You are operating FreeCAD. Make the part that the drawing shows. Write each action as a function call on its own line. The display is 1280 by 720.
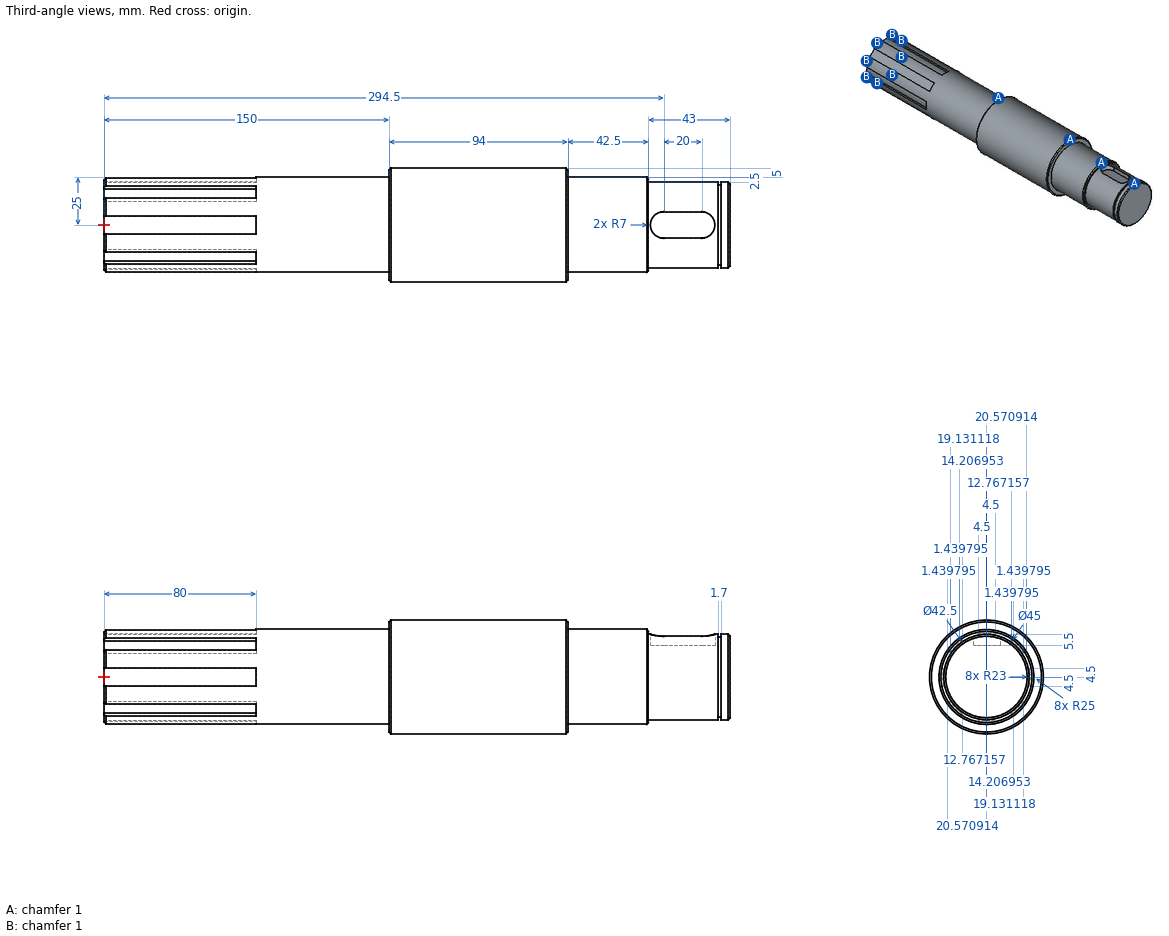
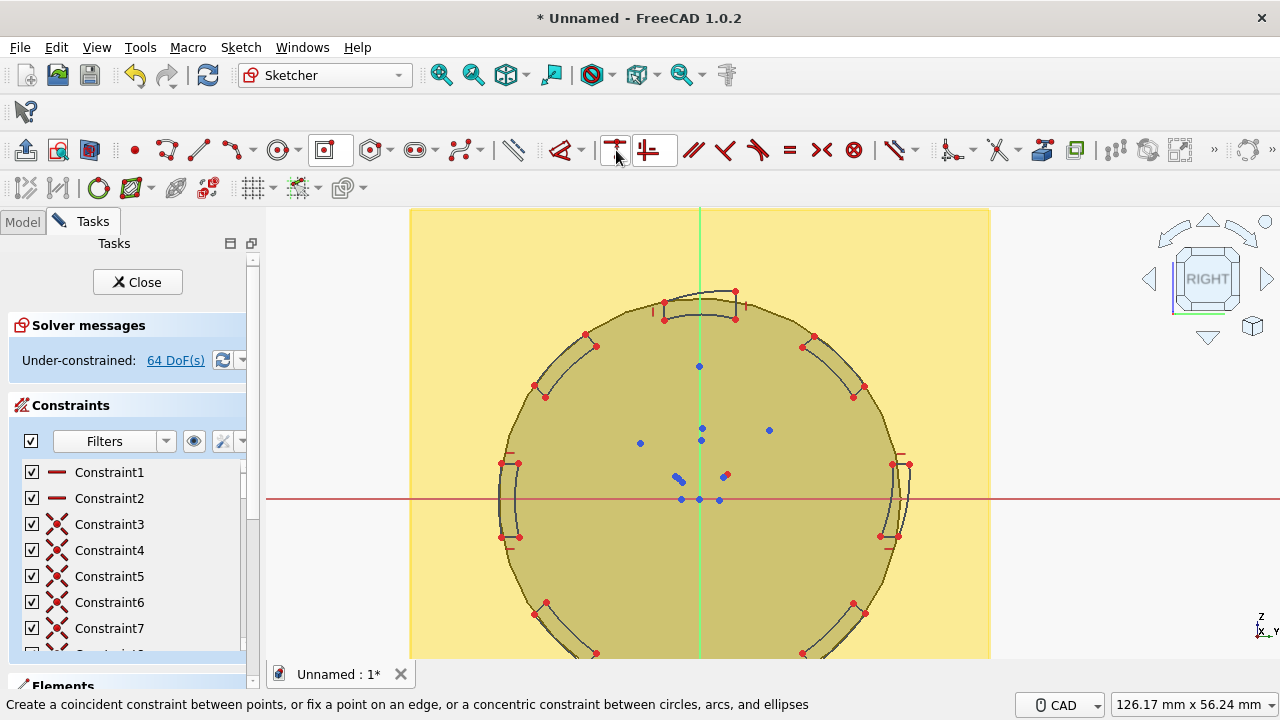
click(888, 516)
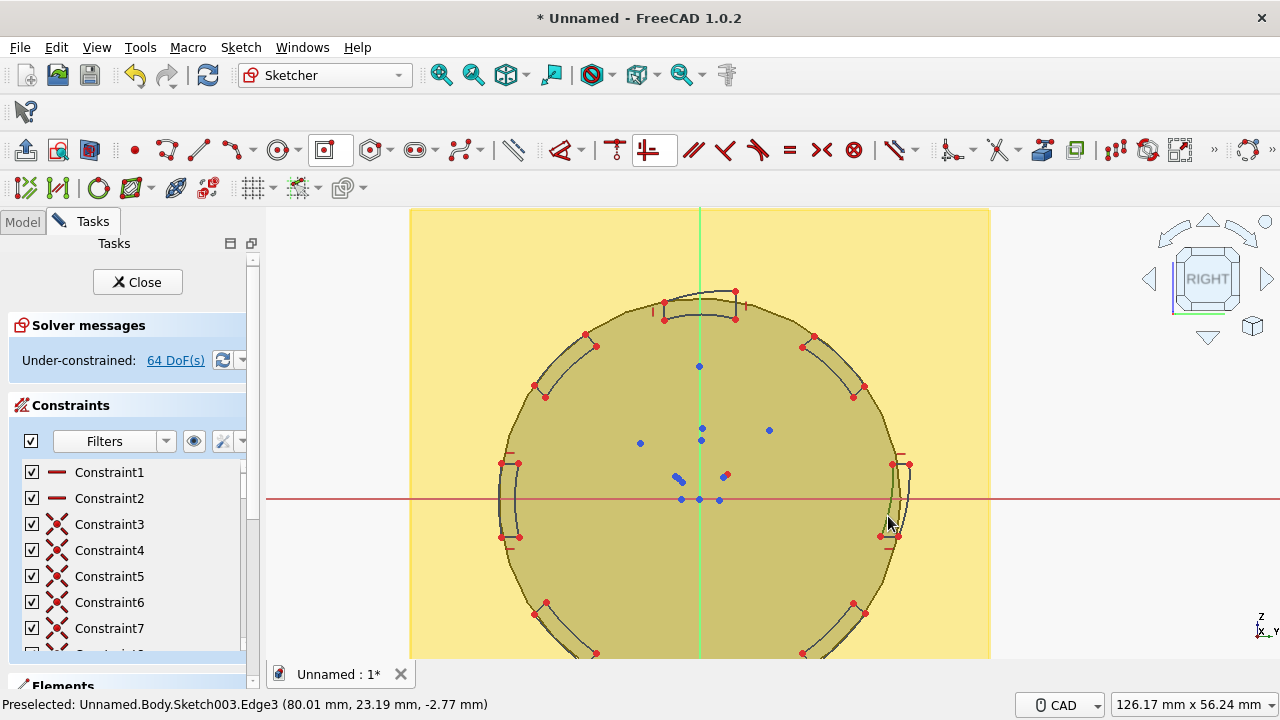
click(714, 315)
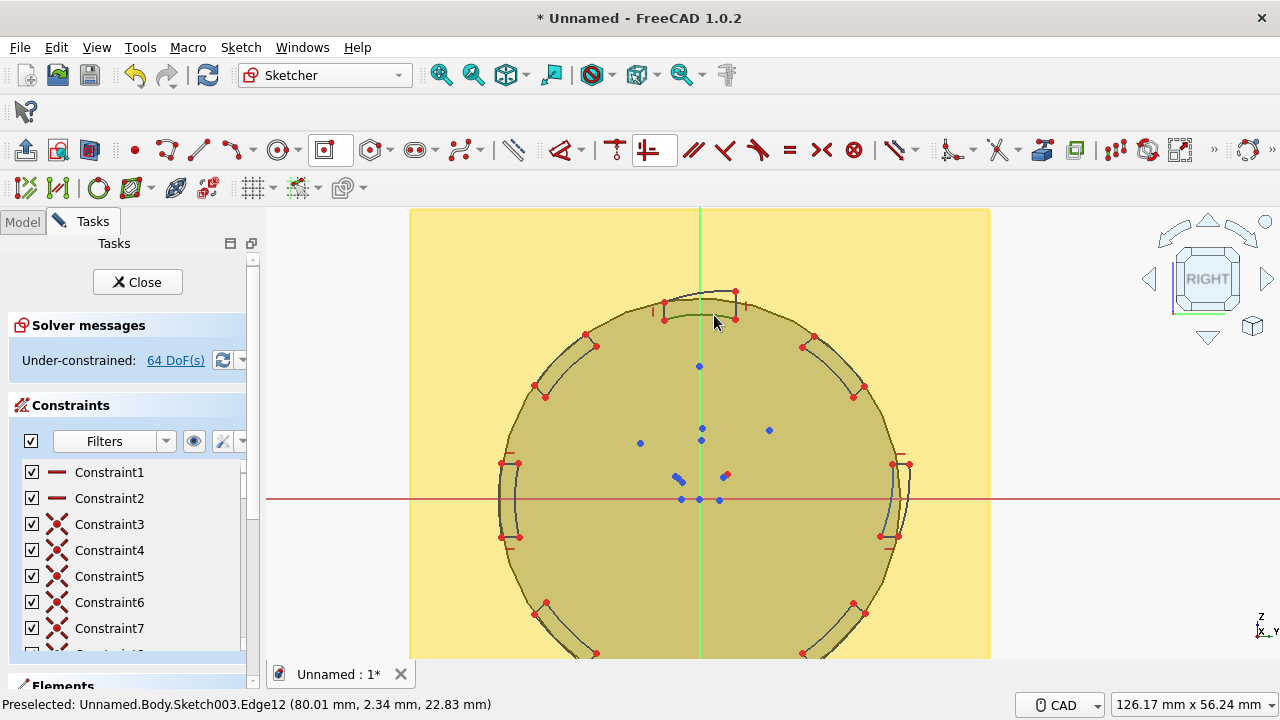
click(616, 150)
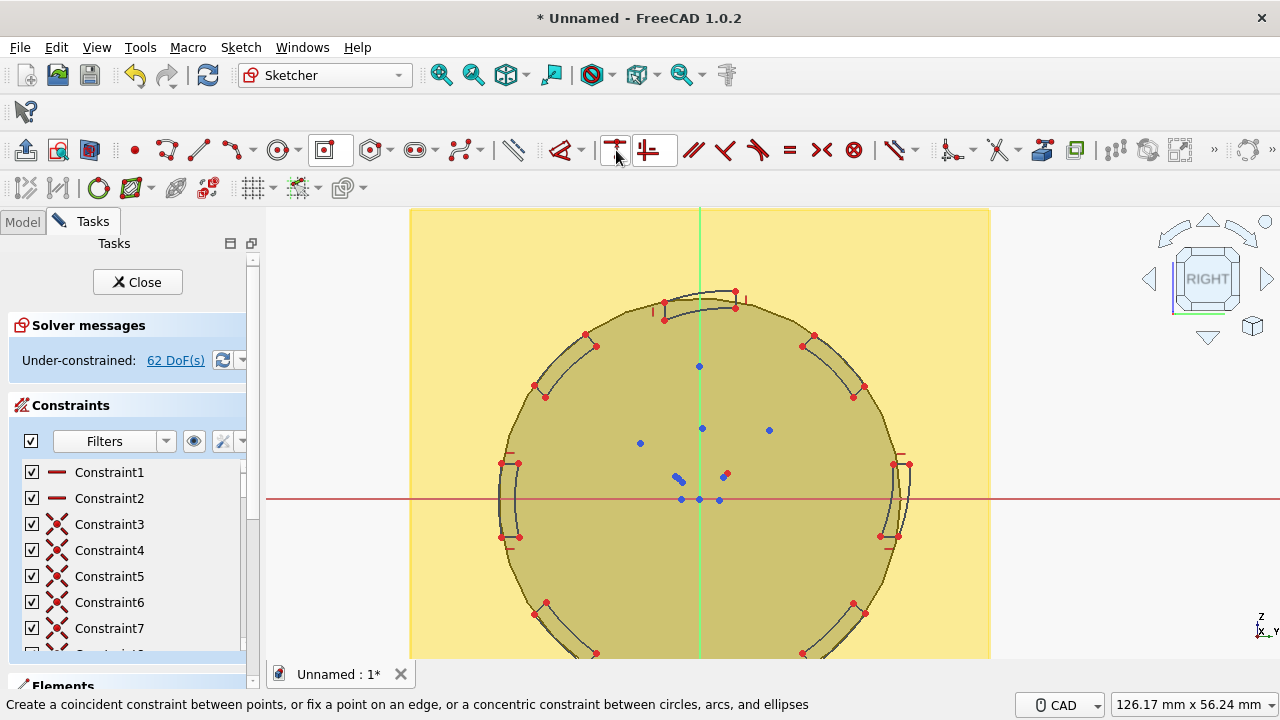
click(888, 516)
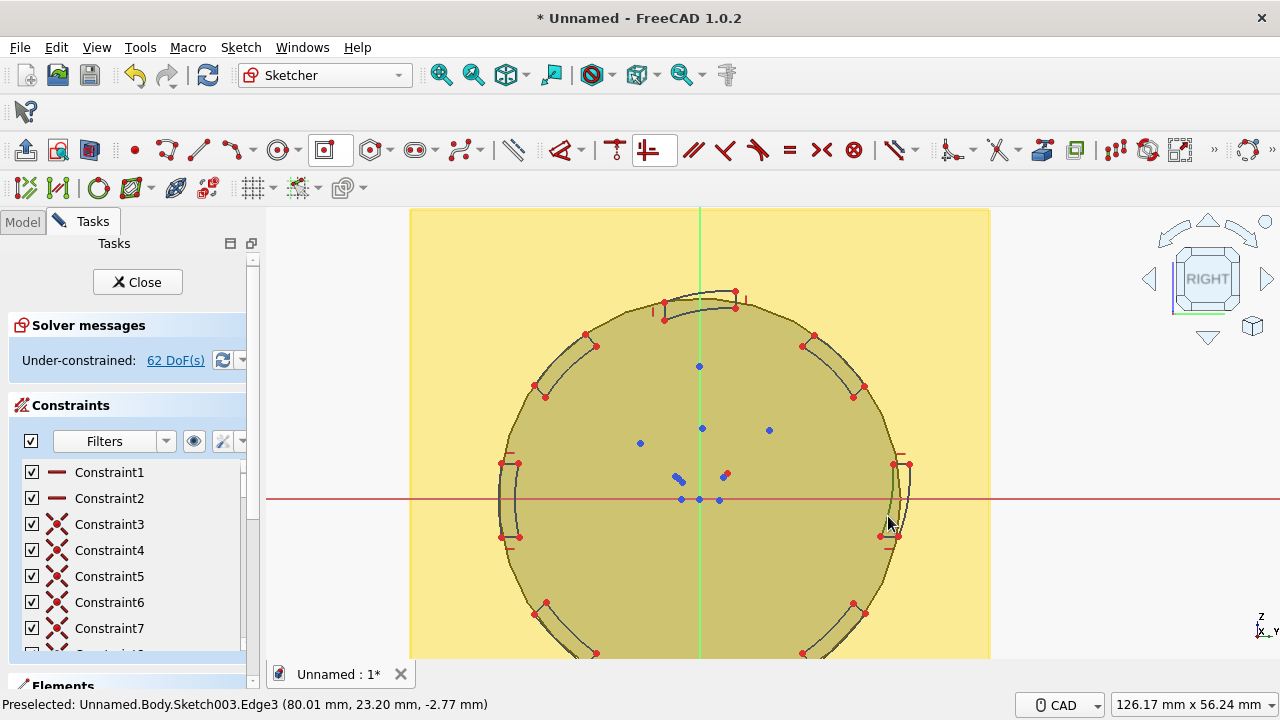
click(568, 347)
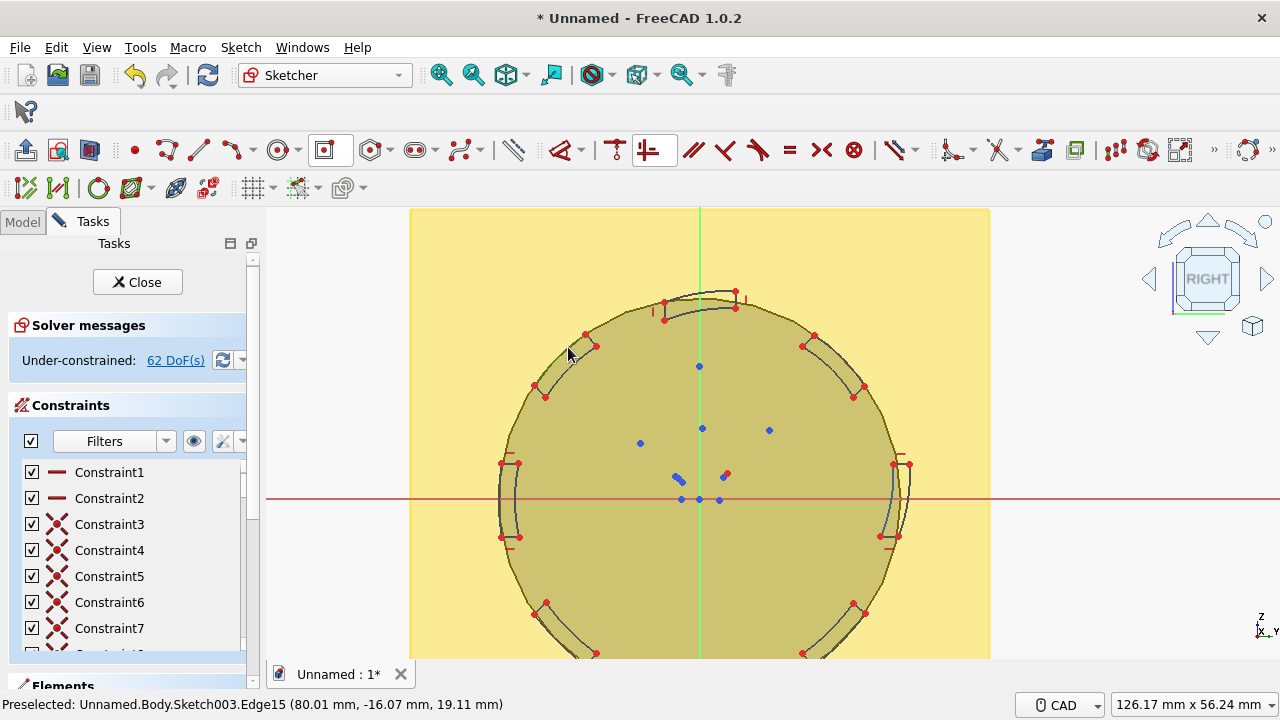
click(616, 150)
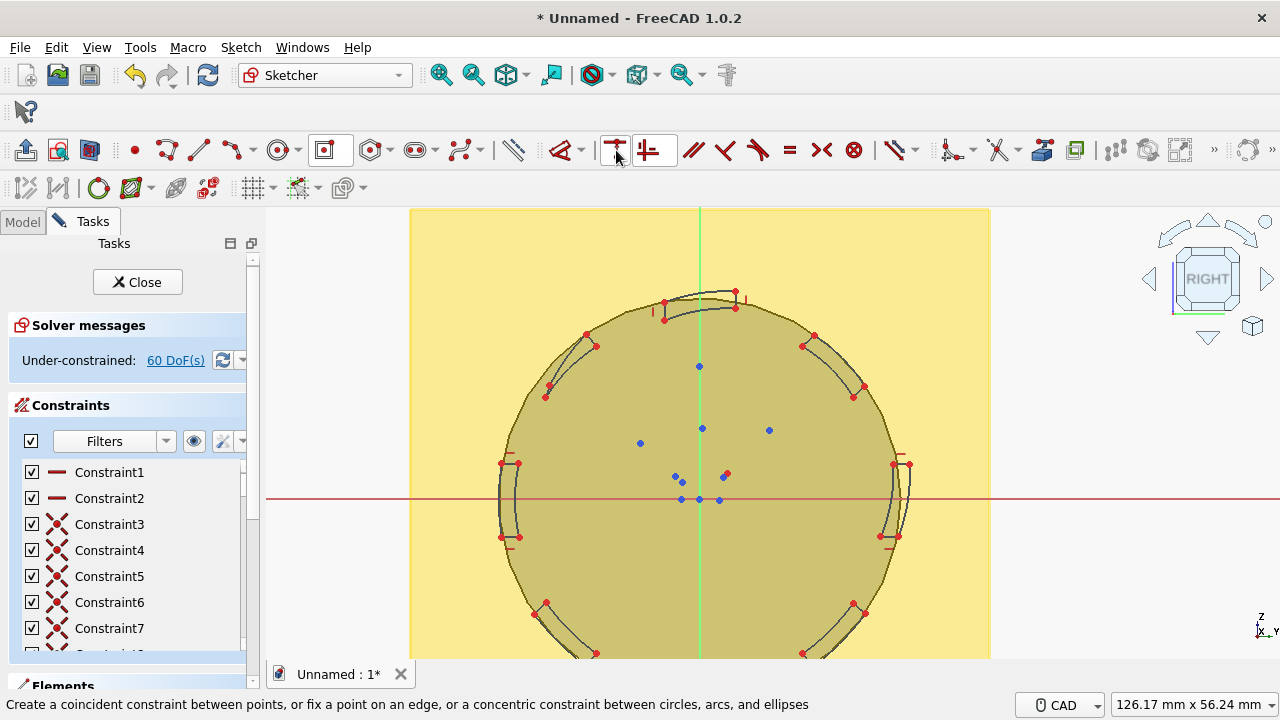
click(888, 516)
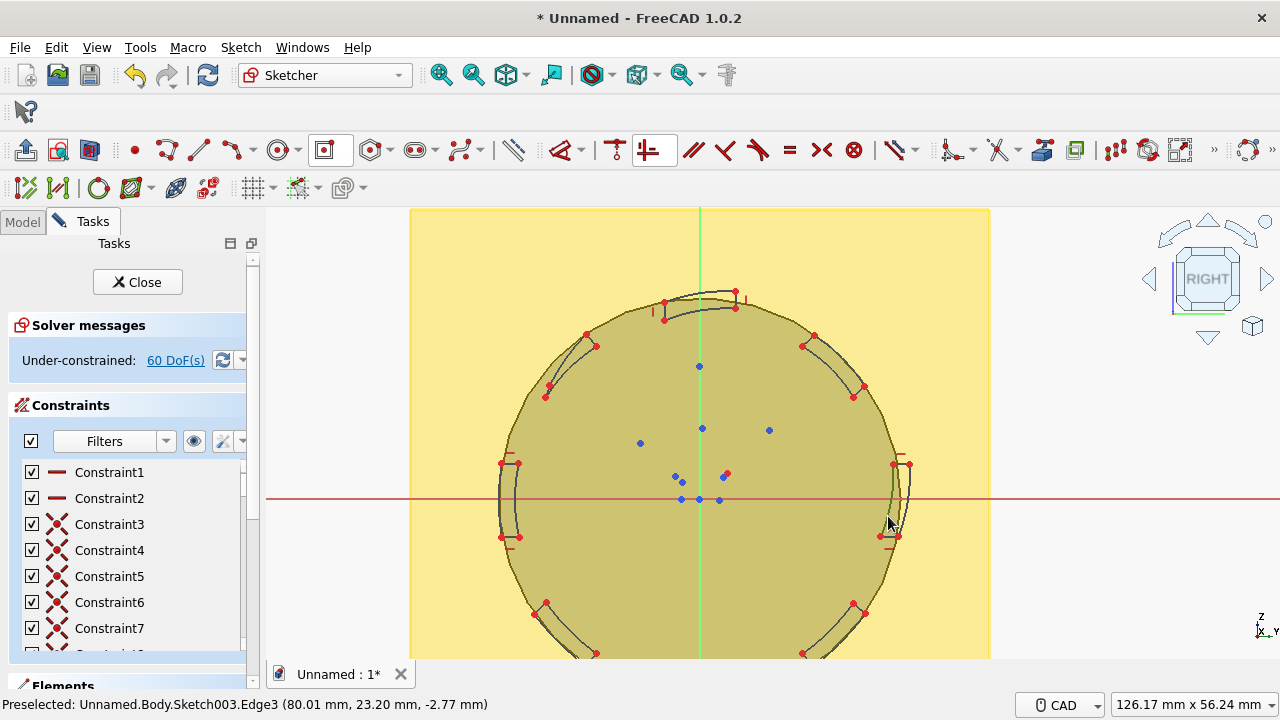
scroll(579, 359, up, 2)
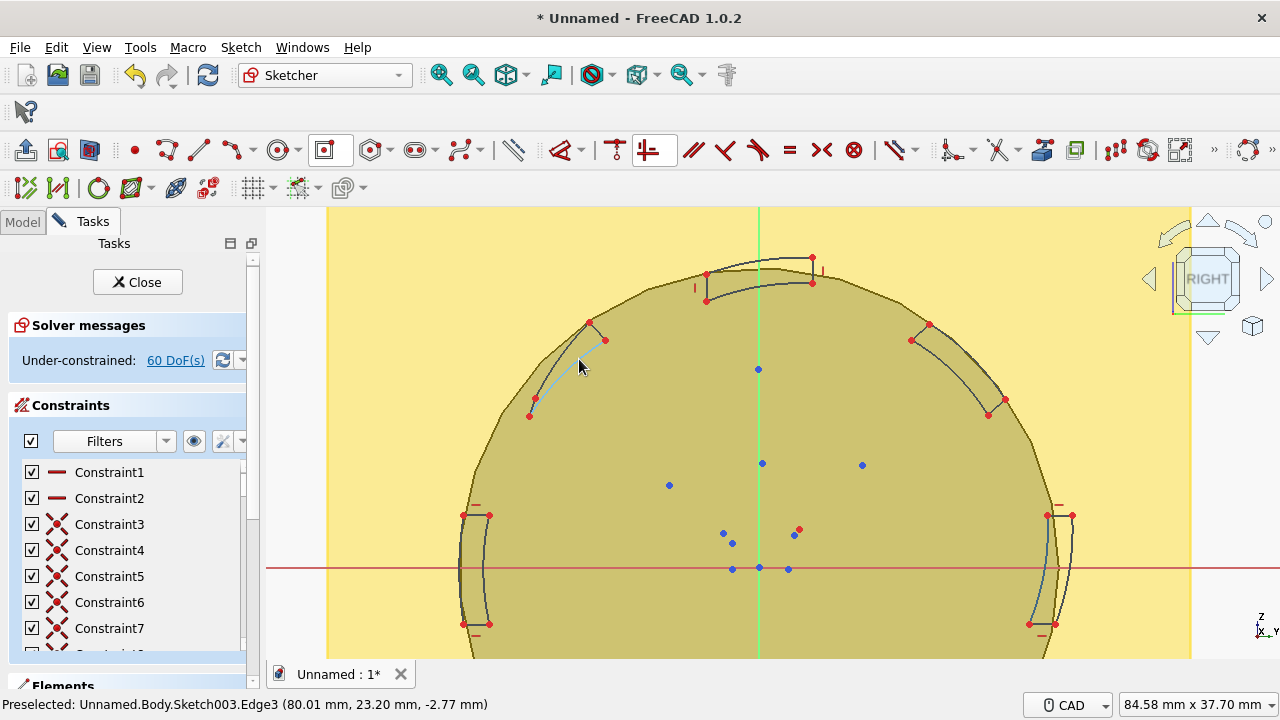
click(579, 359)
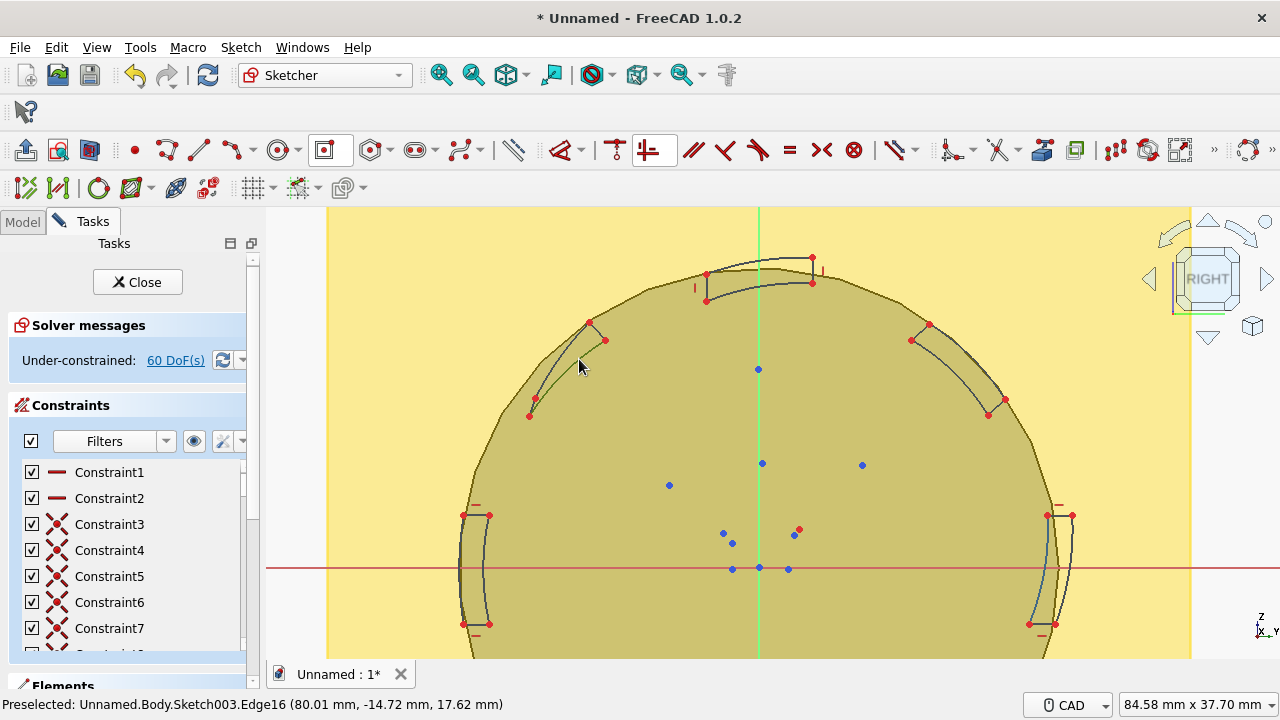
click(616, 150)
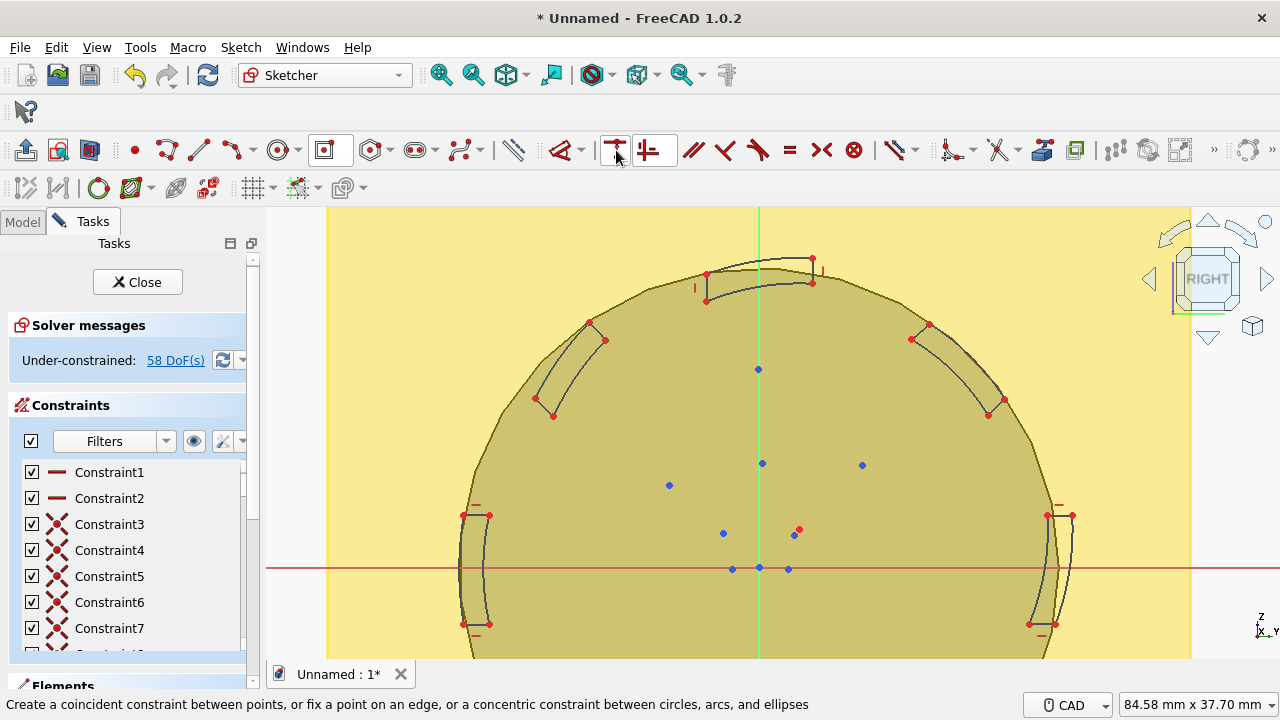
click(1040, 593)